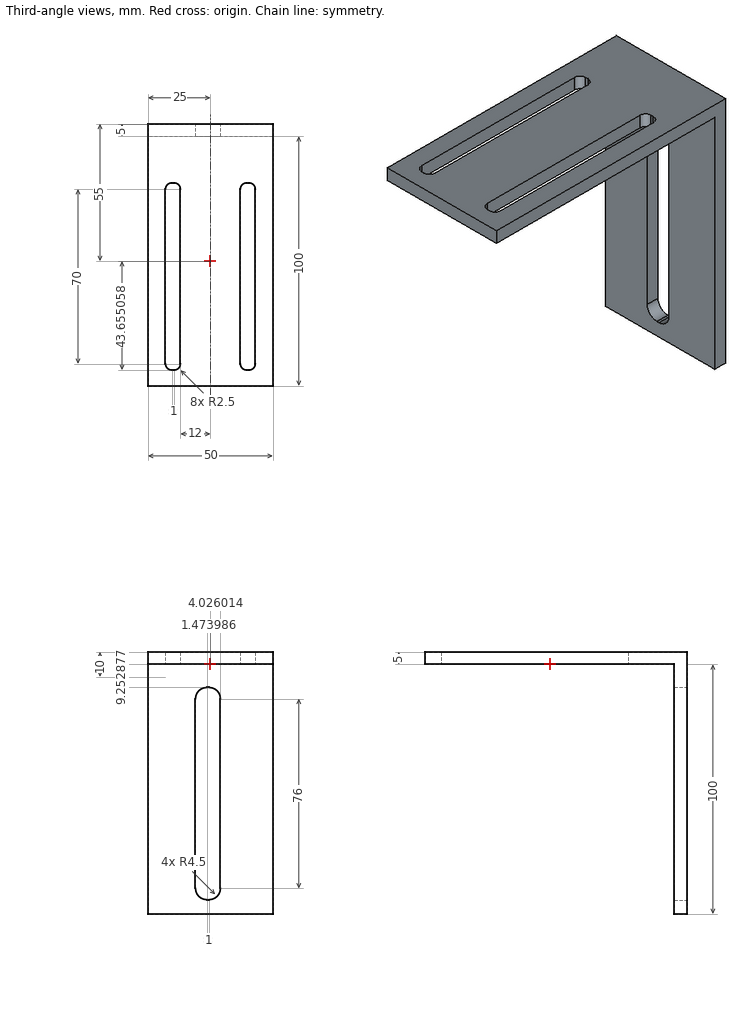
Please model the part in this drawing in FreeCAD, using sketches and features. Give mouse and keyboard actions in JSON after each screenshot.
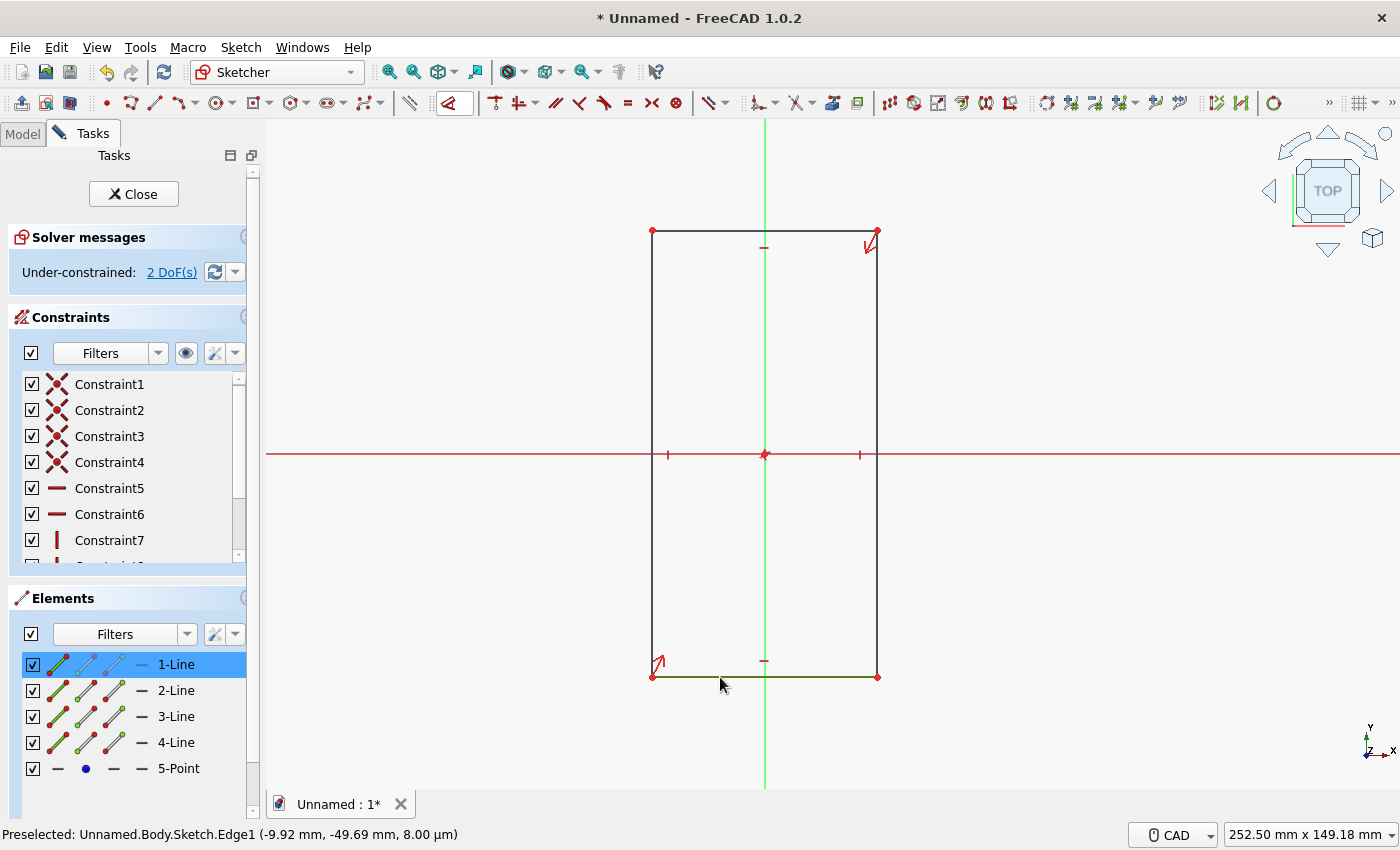
{"action": "left_click", "coordinate": [468, 104]}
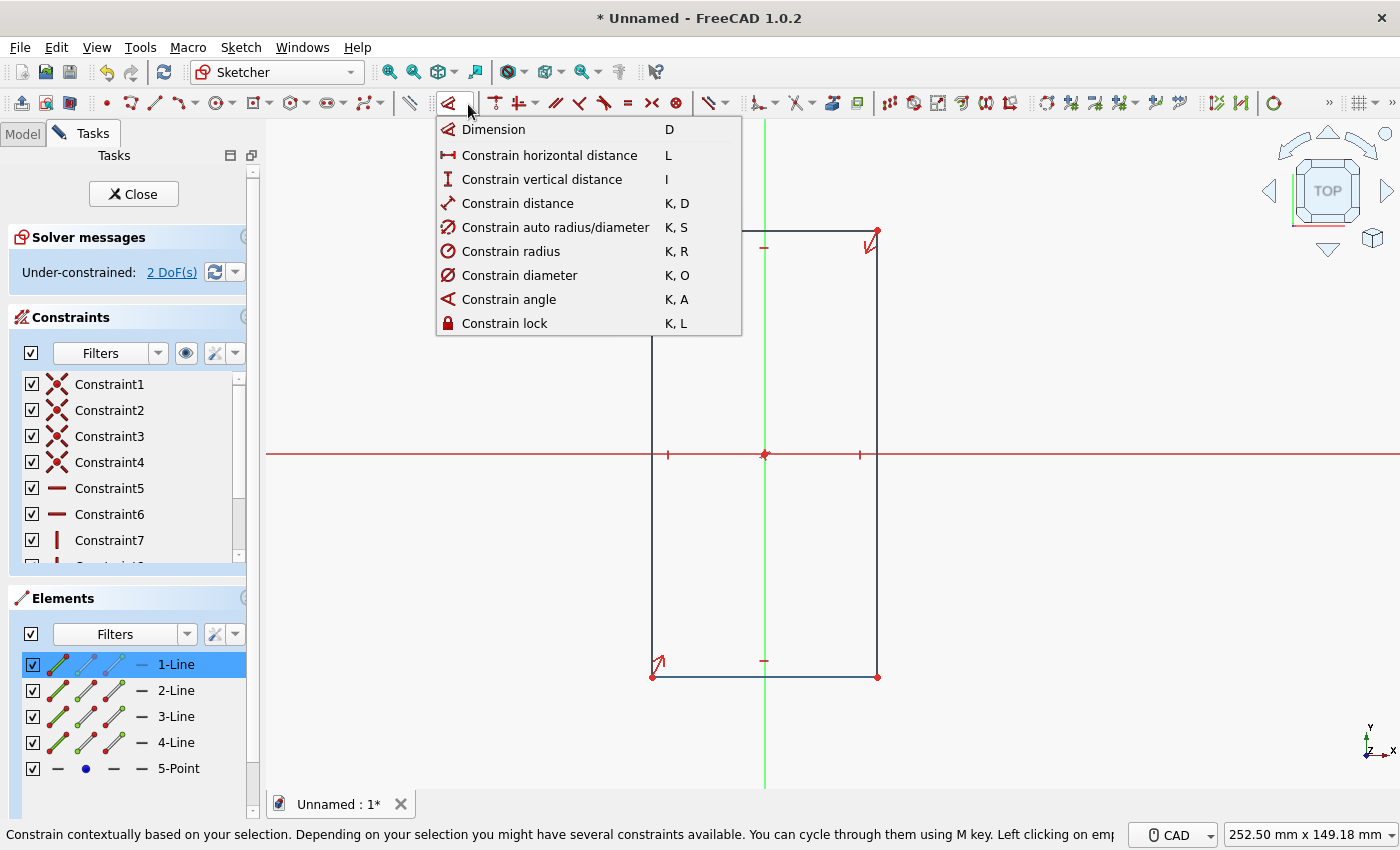
{"action": "left_click", "coordinate": [589, 155]}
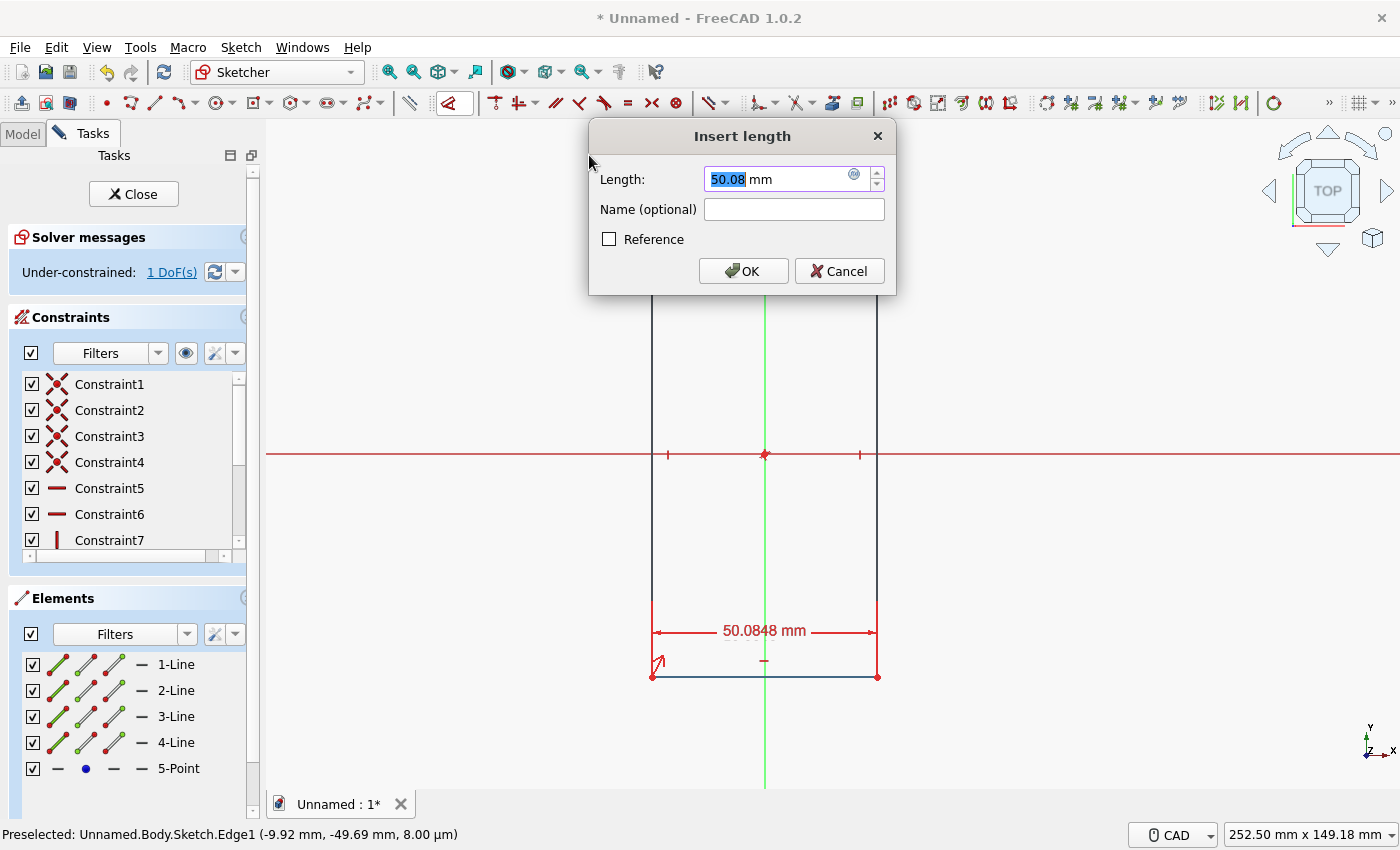
{"action": "type", "text": "50"}
{"action": "key", "text": "Return"}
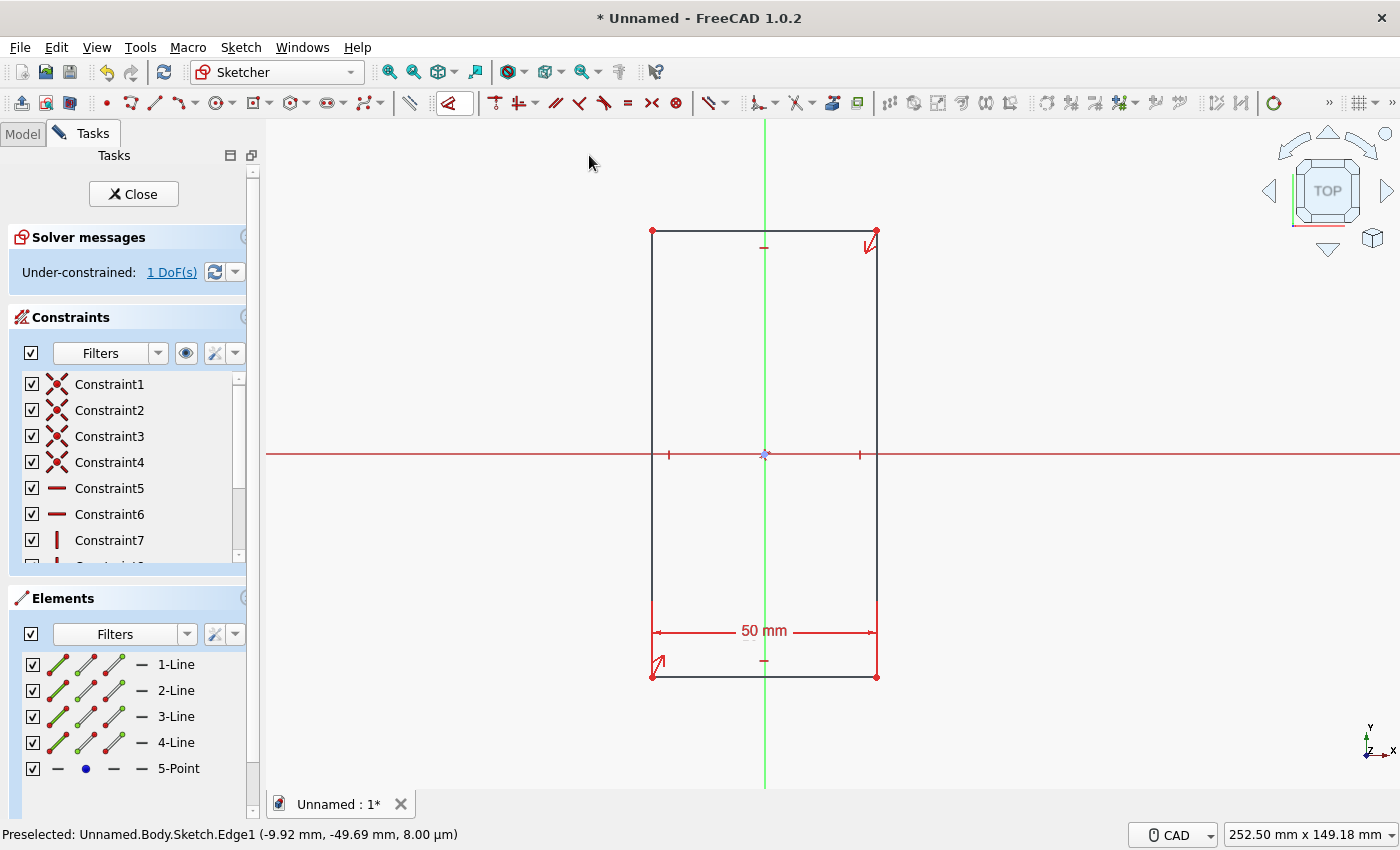
{"action": "left_click", "coordinate": [877, 543]}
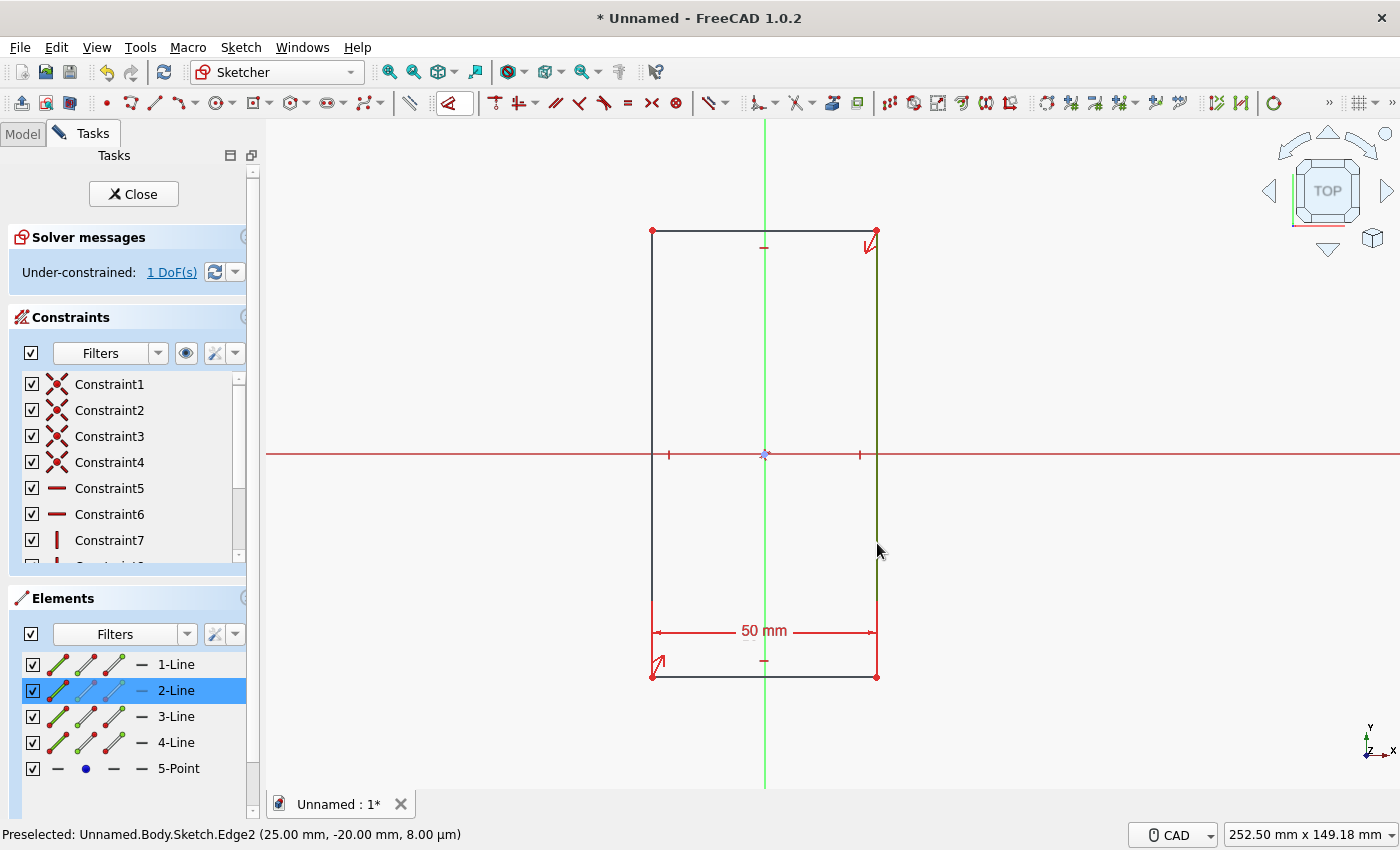
{"action": "key", "text": "i"}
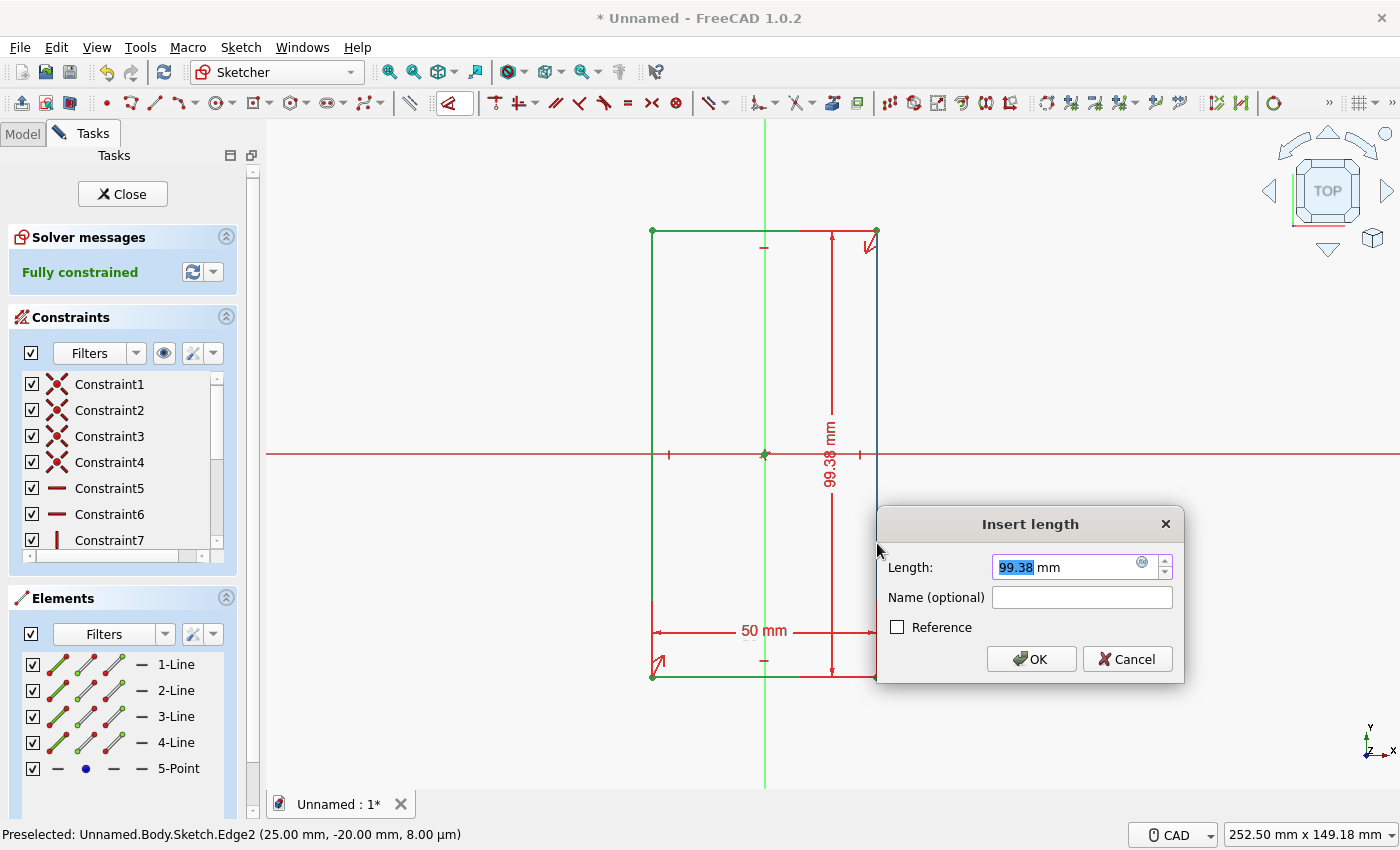
{"action": "type", "text": "100"}
{"action": "key", "text": "Return"}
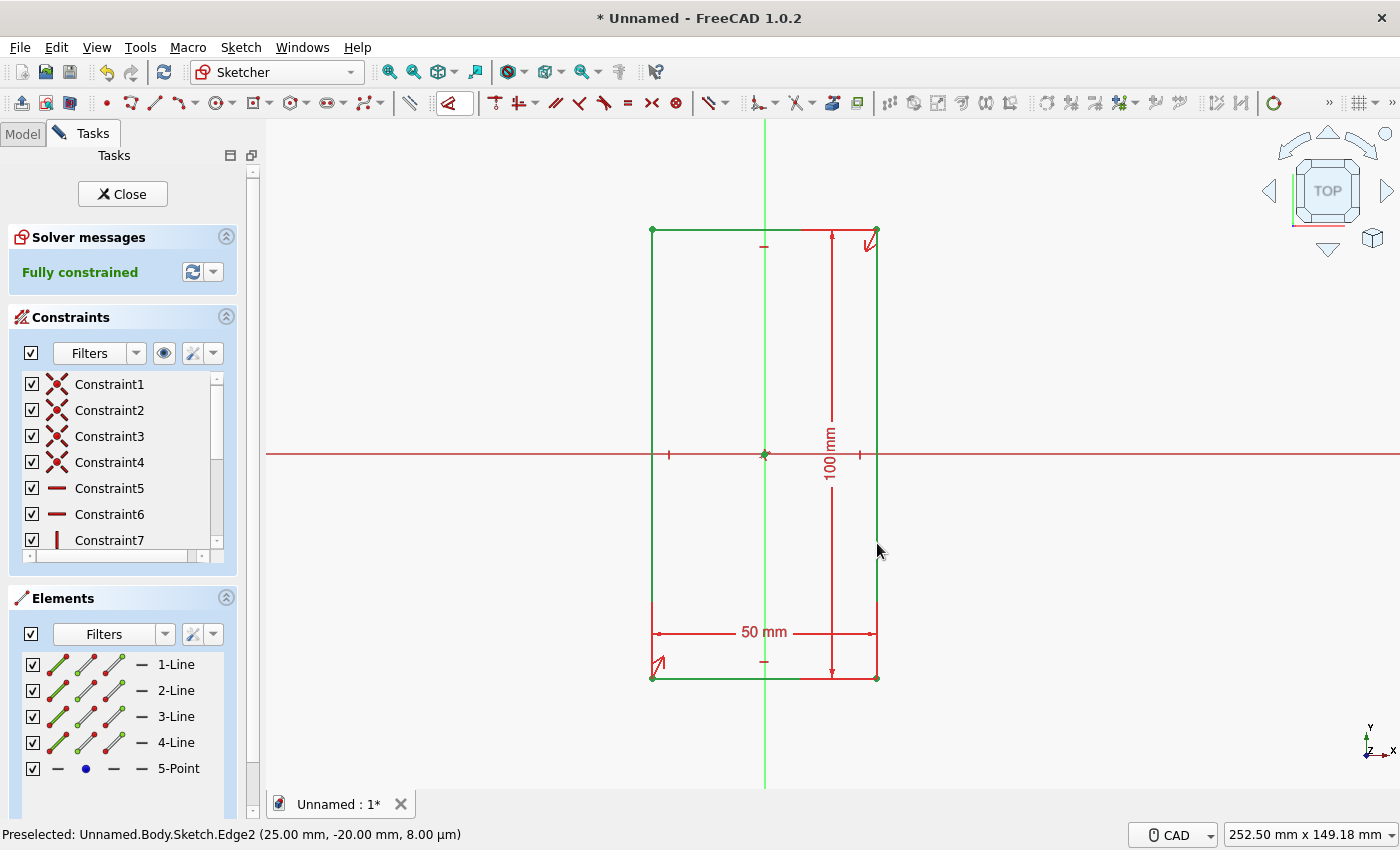
{"action": "left_click", "coordinate": [123, 194]}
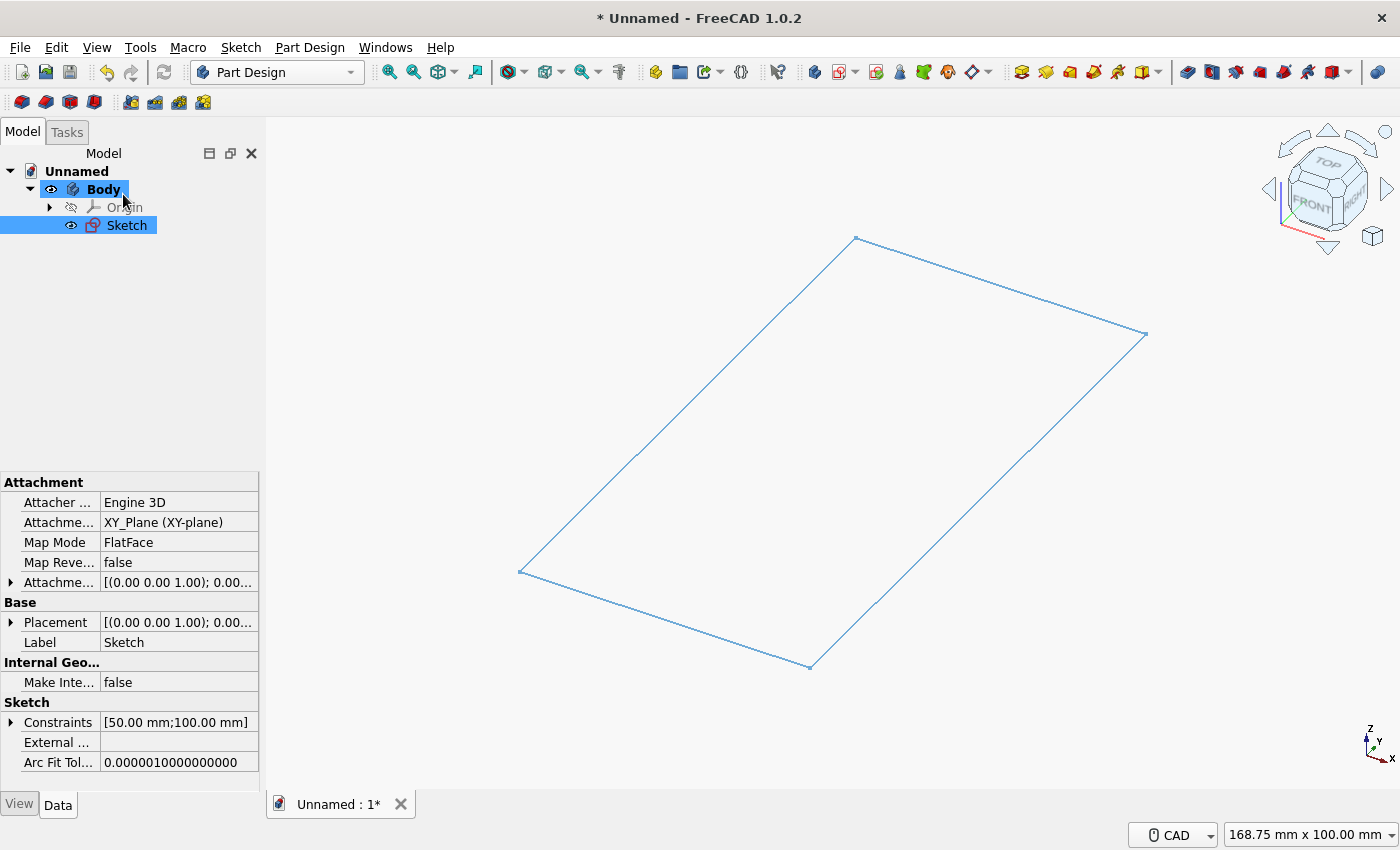
{"action": "left_click", "coordinate": [1022, 72]}